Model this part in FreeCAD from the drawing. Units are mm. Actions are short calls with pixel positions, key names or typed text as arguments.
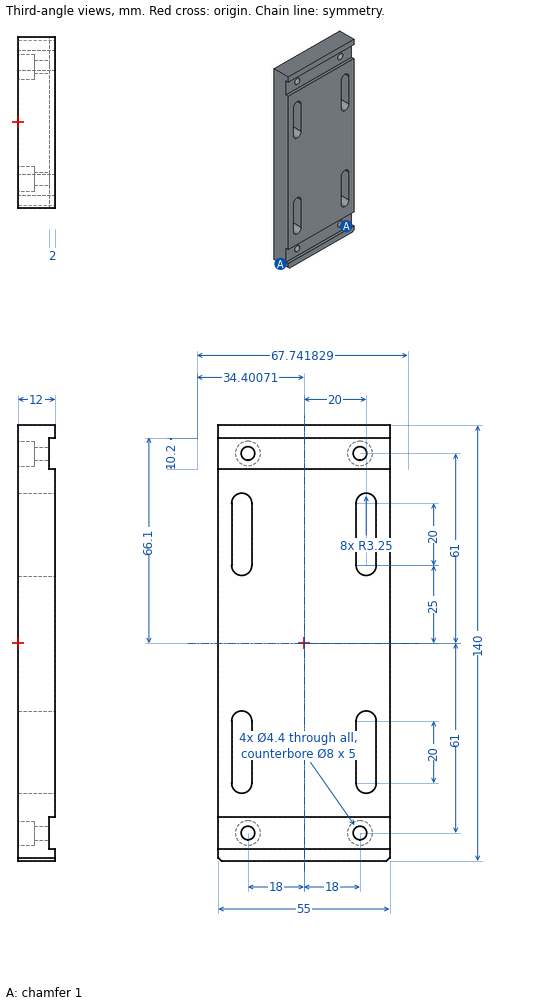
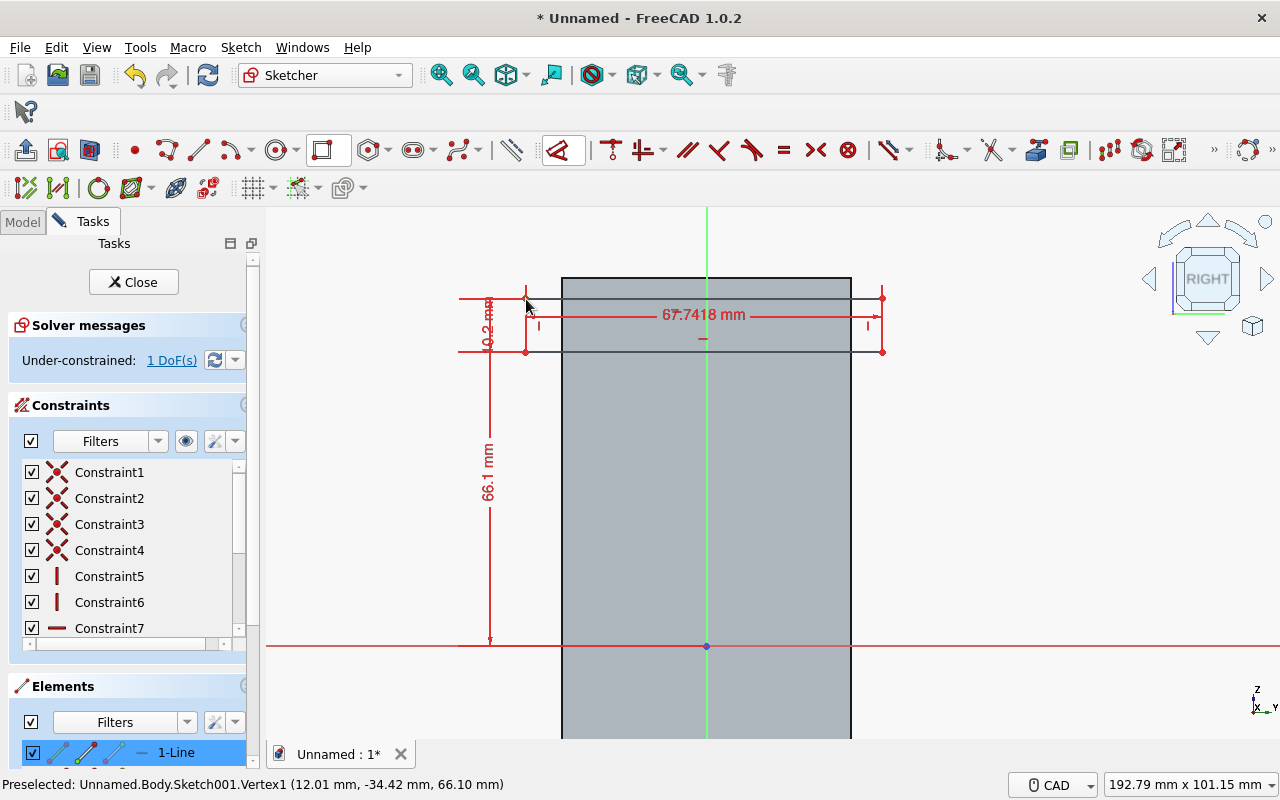
key(l)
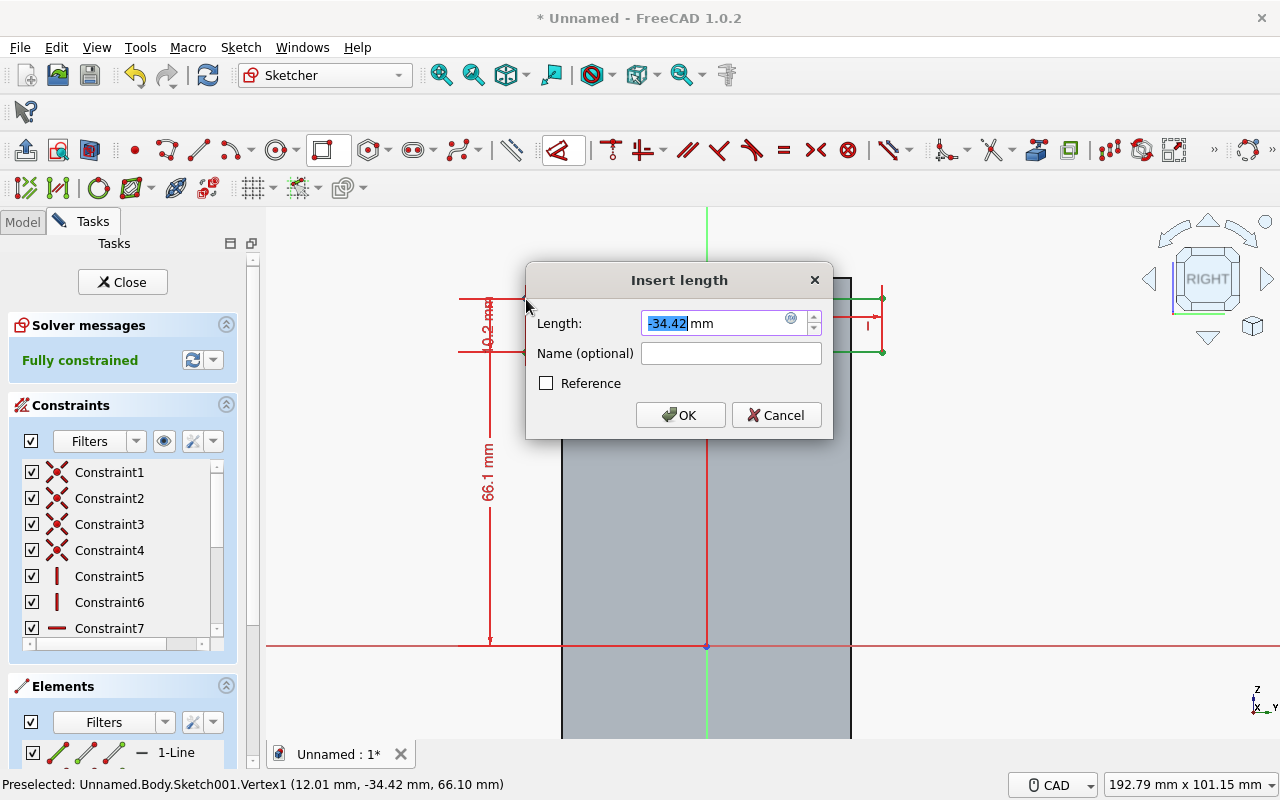
text(-34.40071)
key(Return)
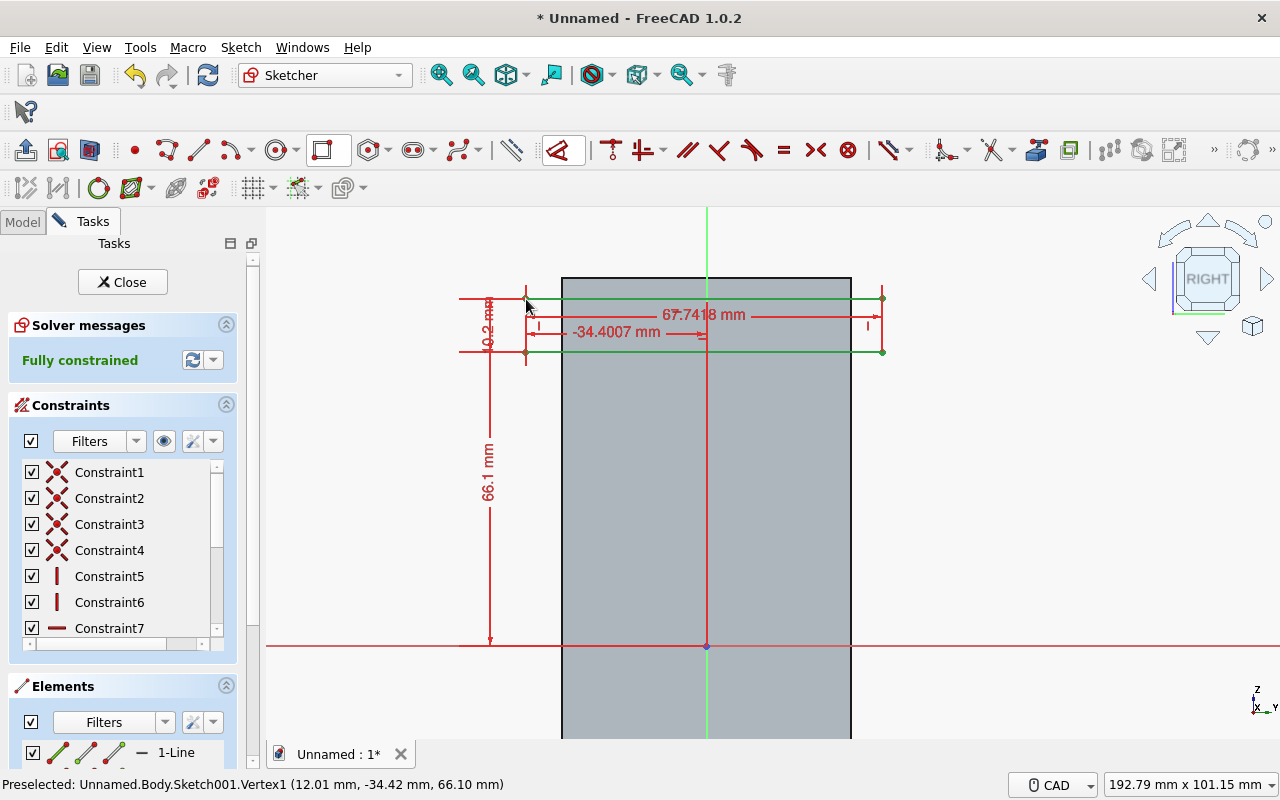
click(123, 282)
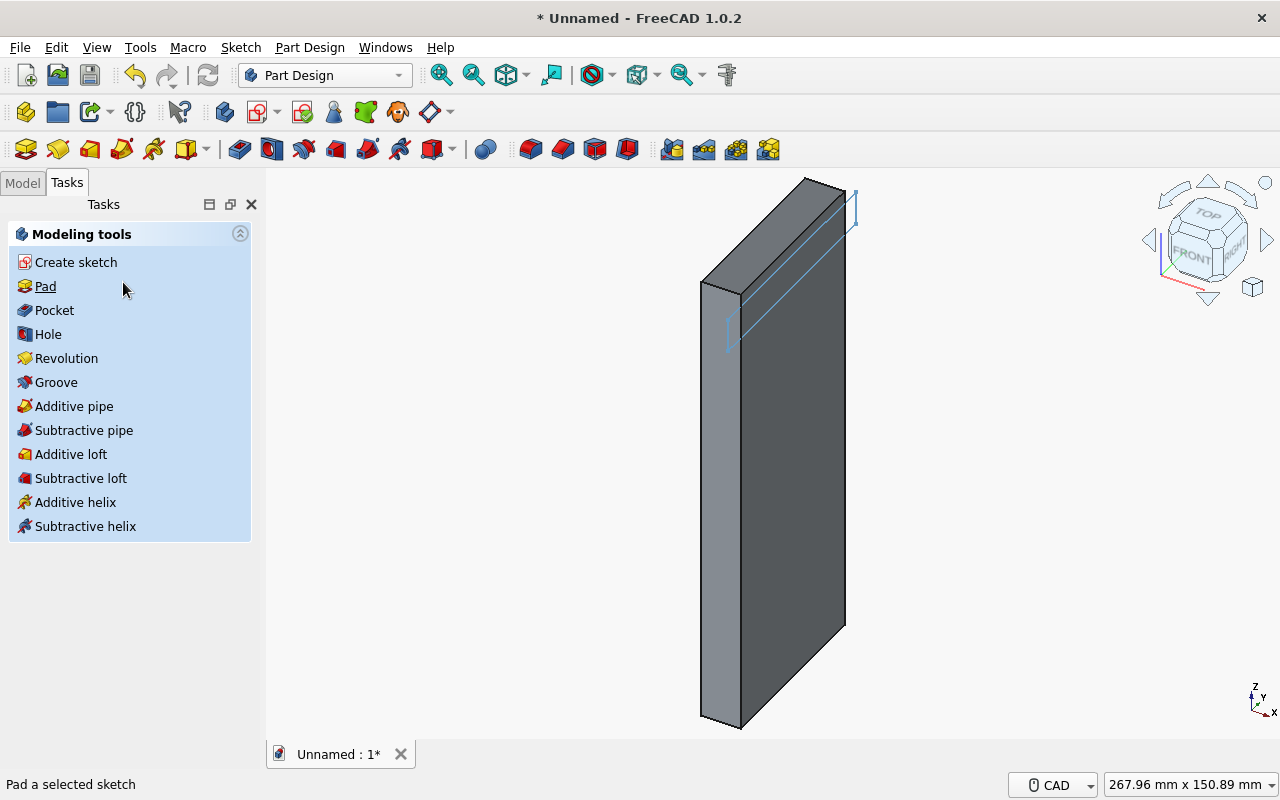
click(240, 150)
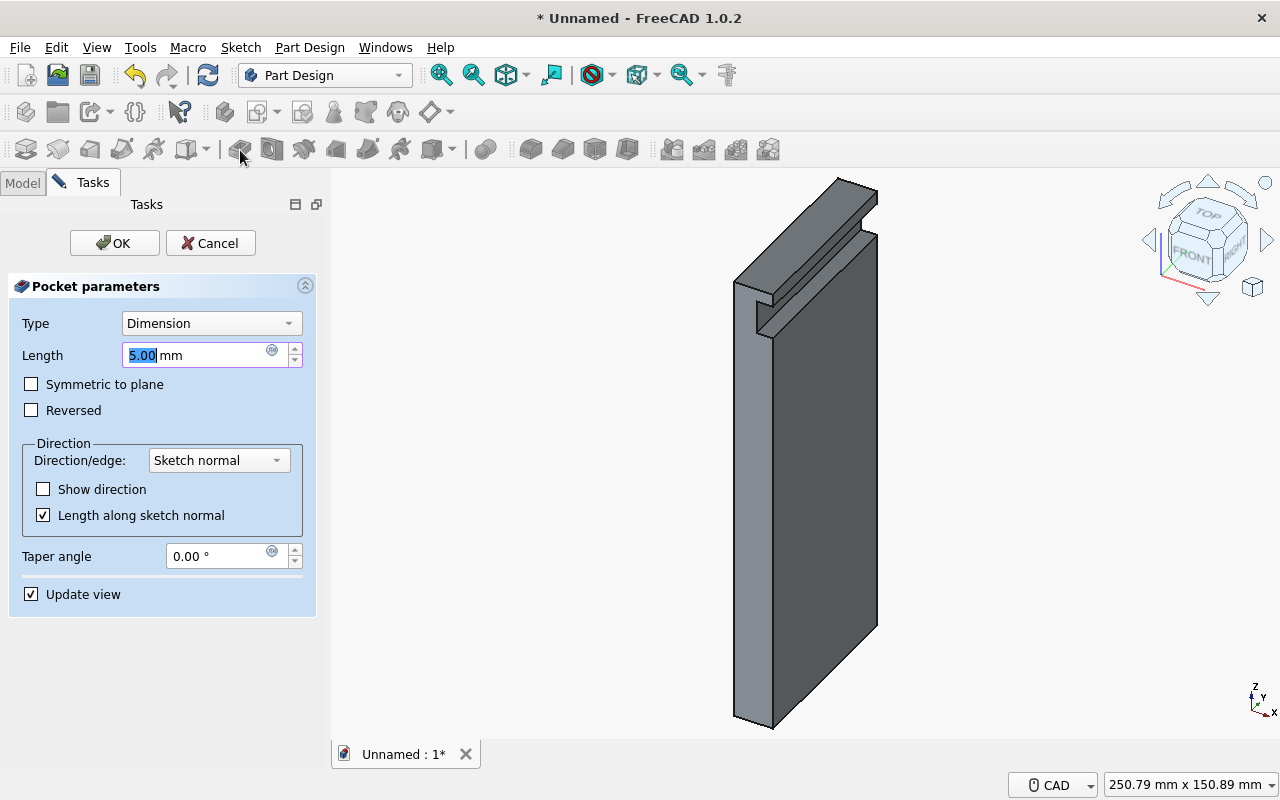
text(2)
key(Tab)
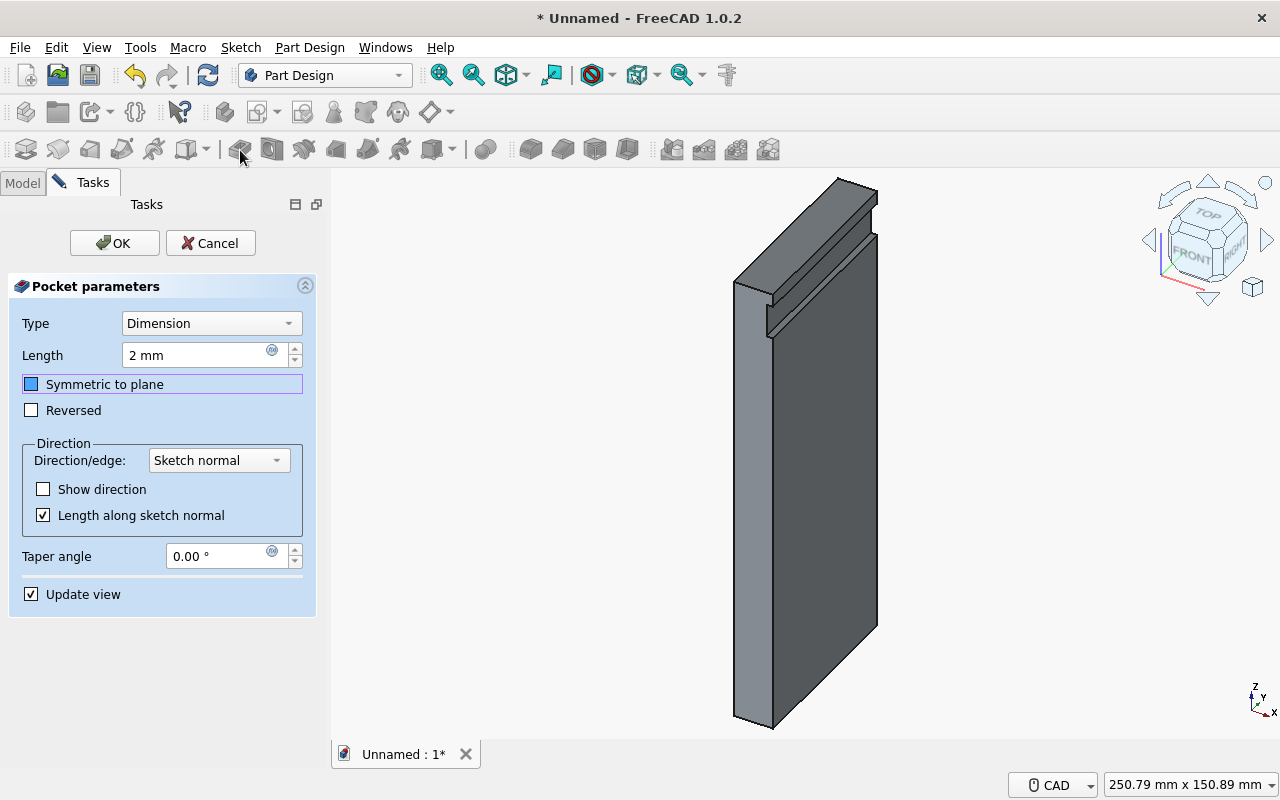
click(115, 243)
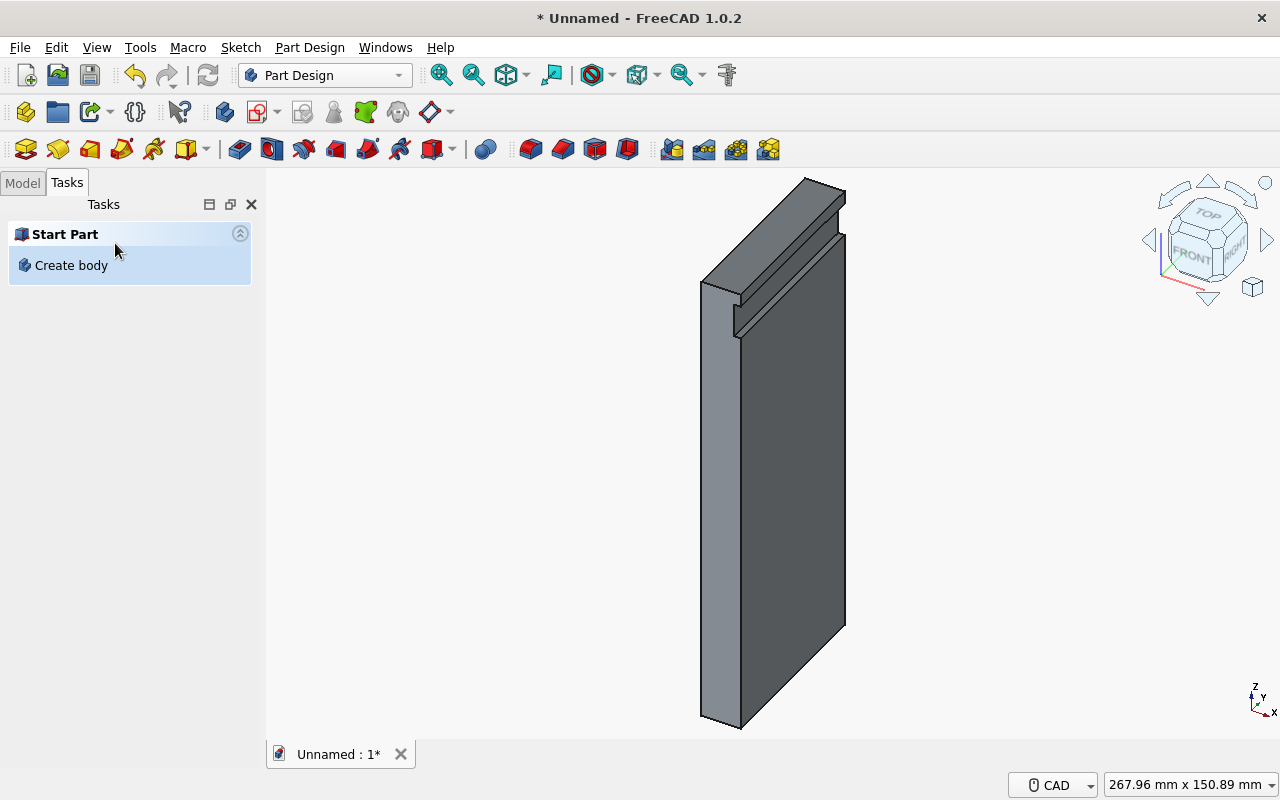
key(0)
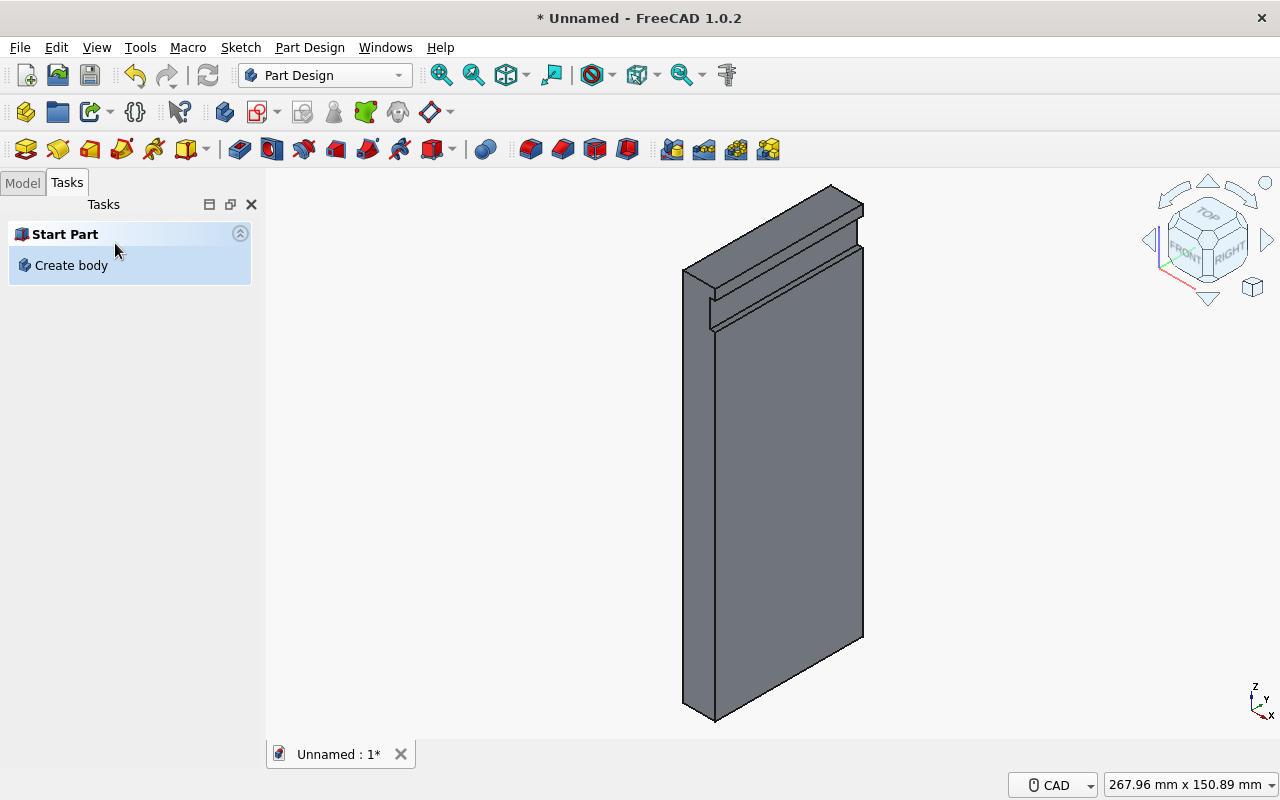
key(2)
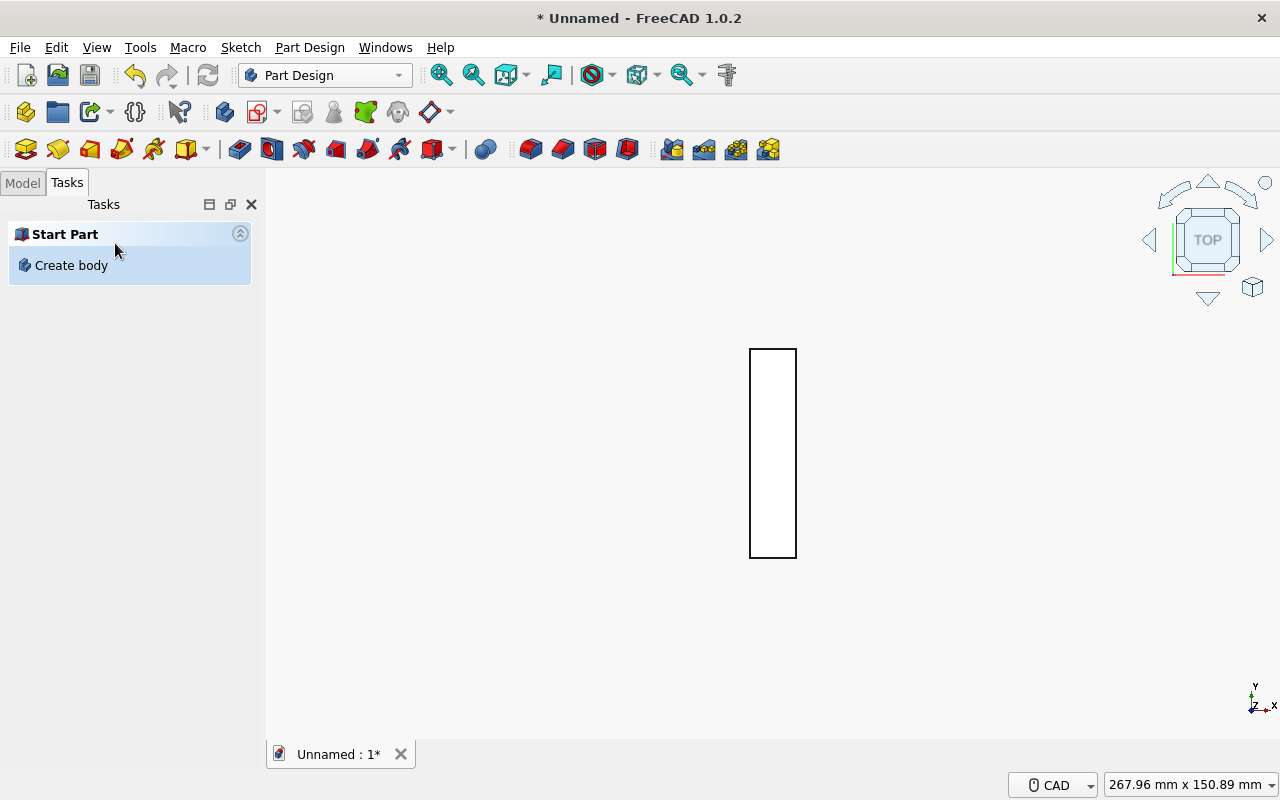
click(442, 76)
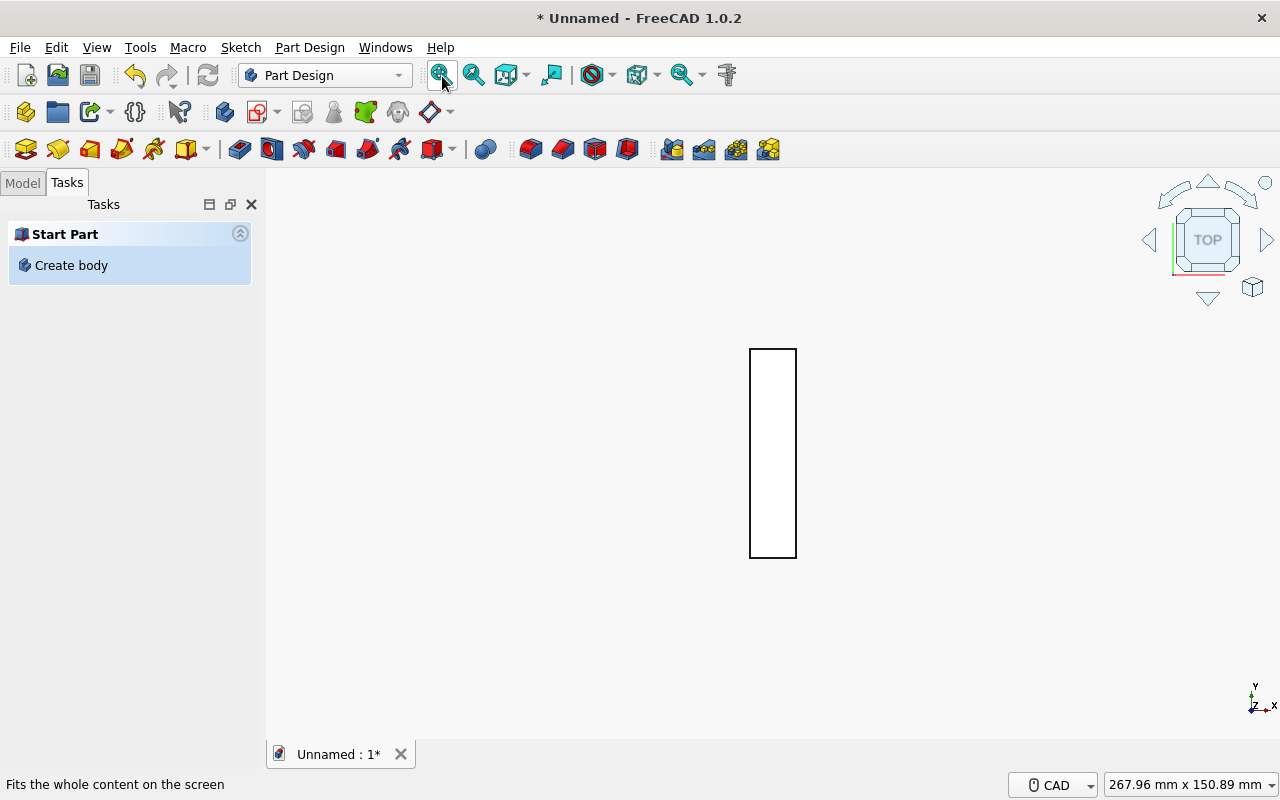
key(1)